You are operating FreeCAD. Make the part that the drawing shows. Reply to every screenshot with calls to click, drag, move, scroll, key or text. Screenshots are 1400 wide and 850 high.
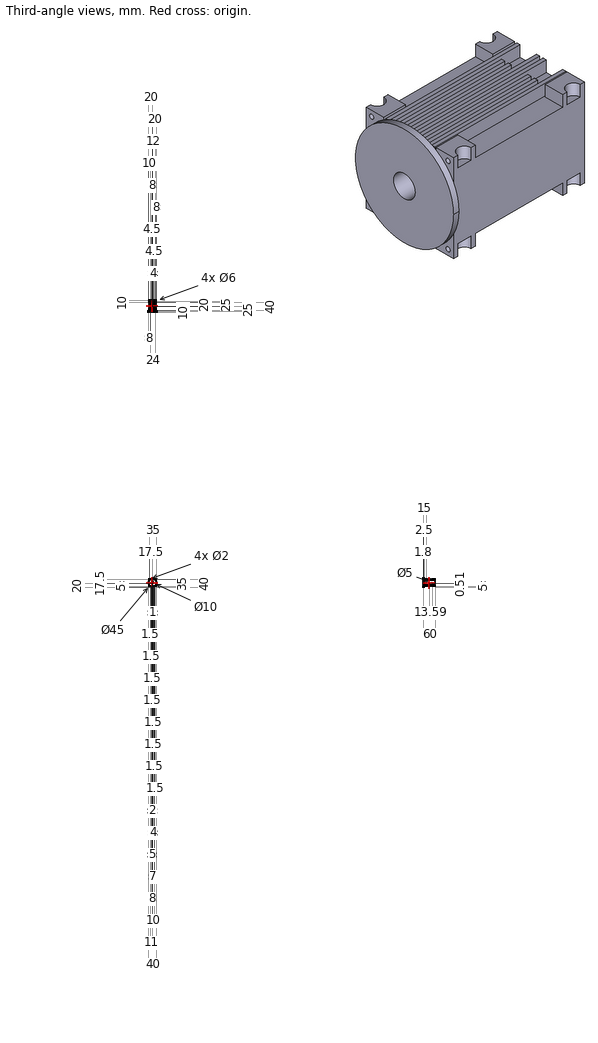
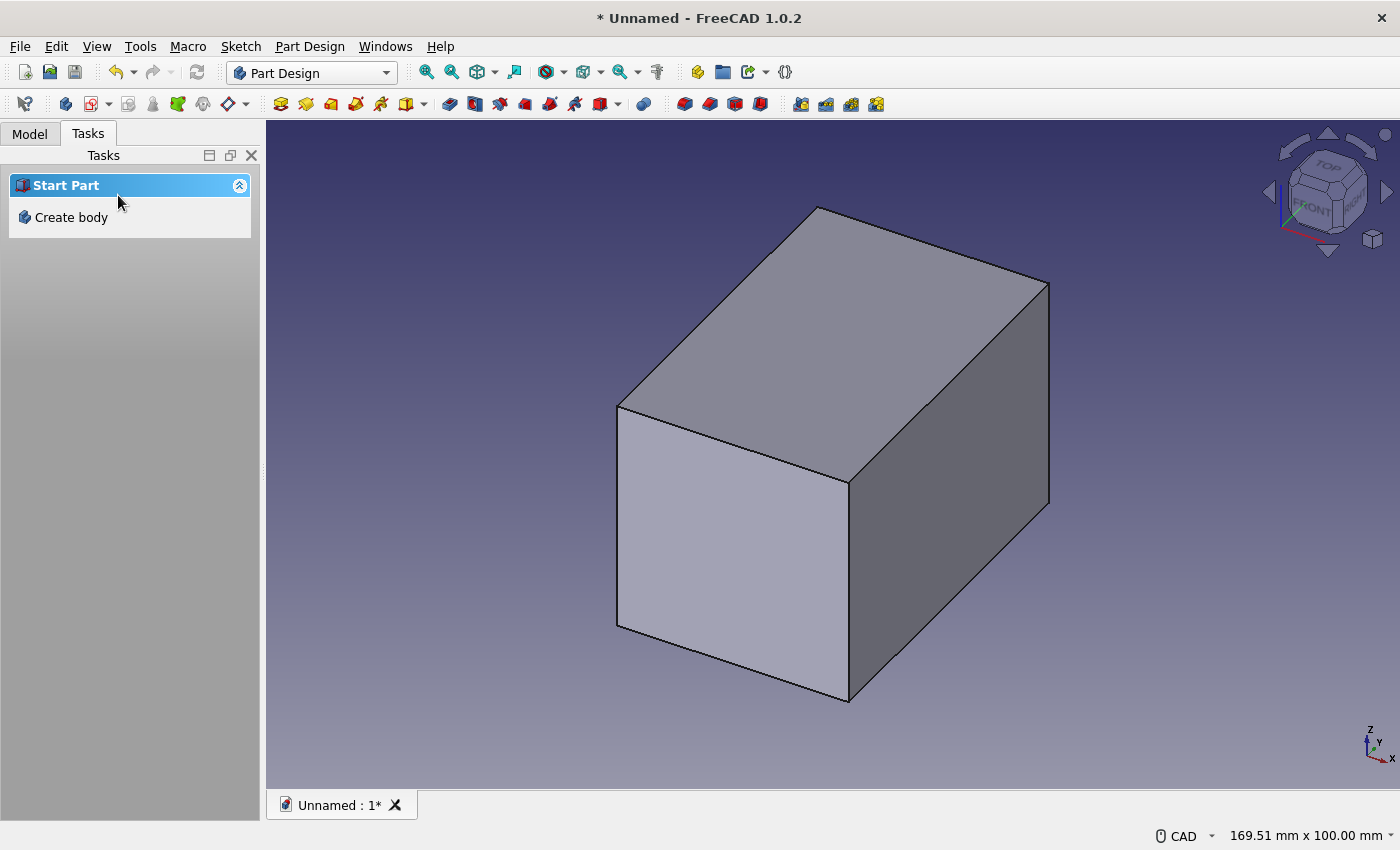
key(5)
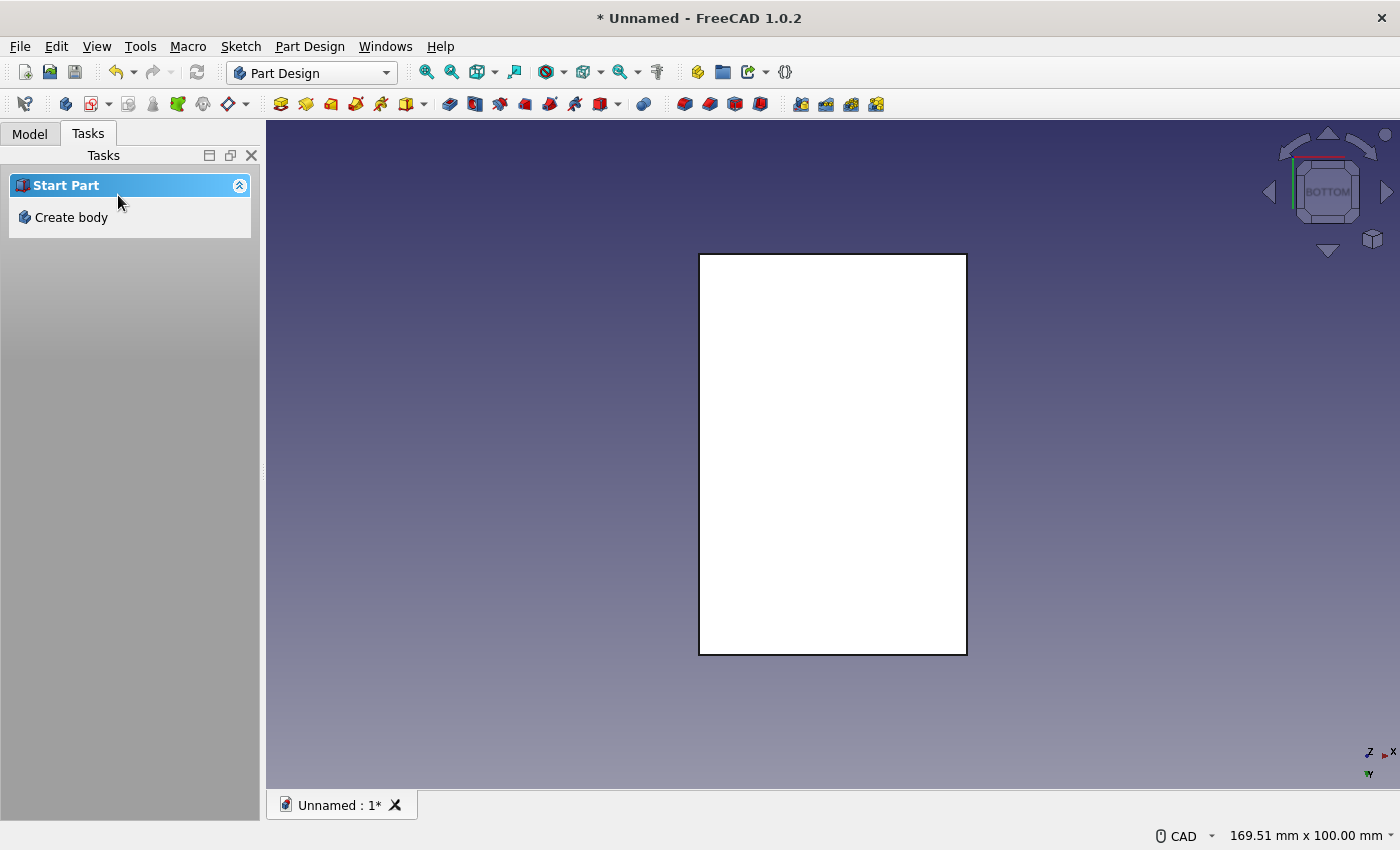
click(833, 511)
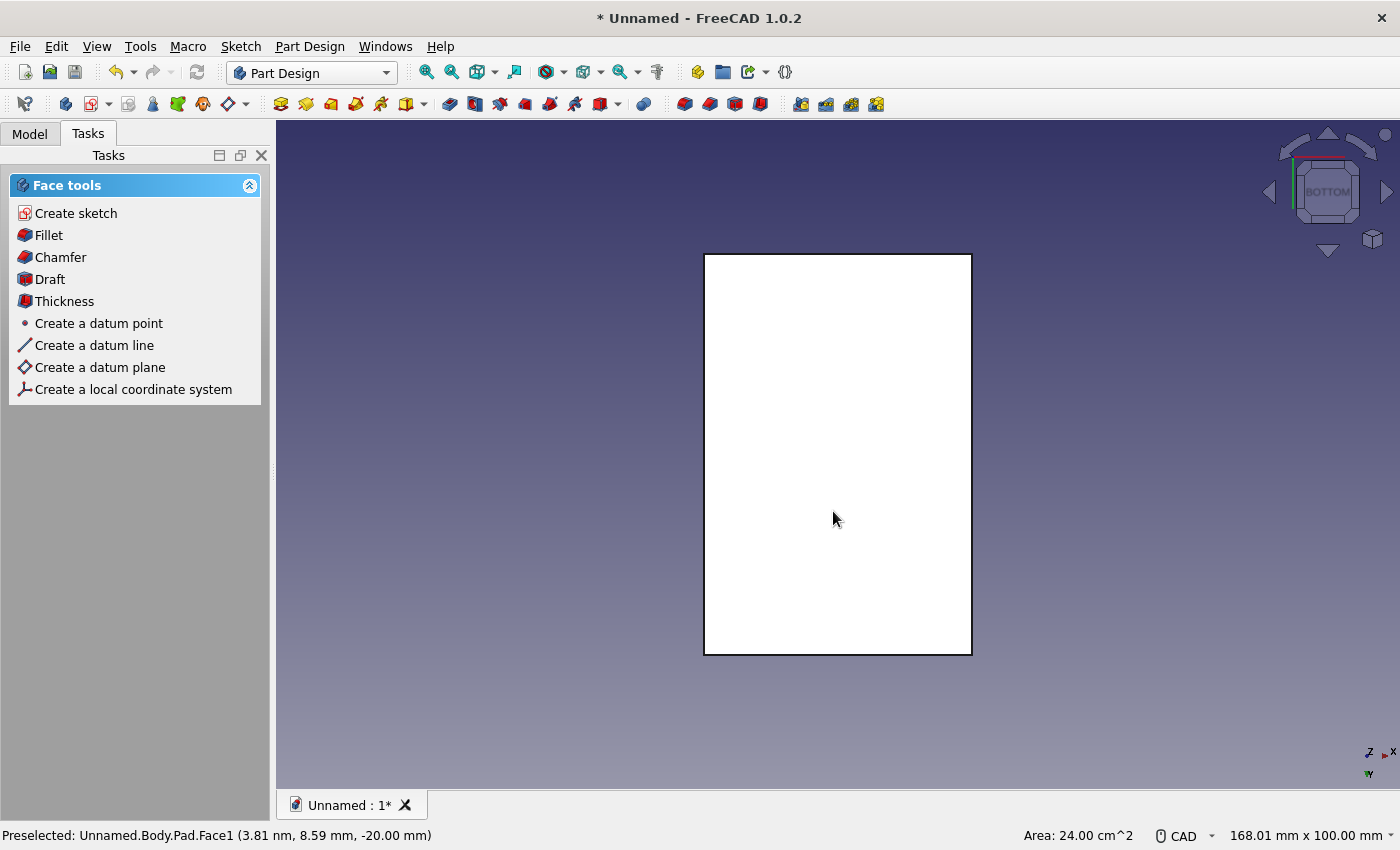
click(90, 104)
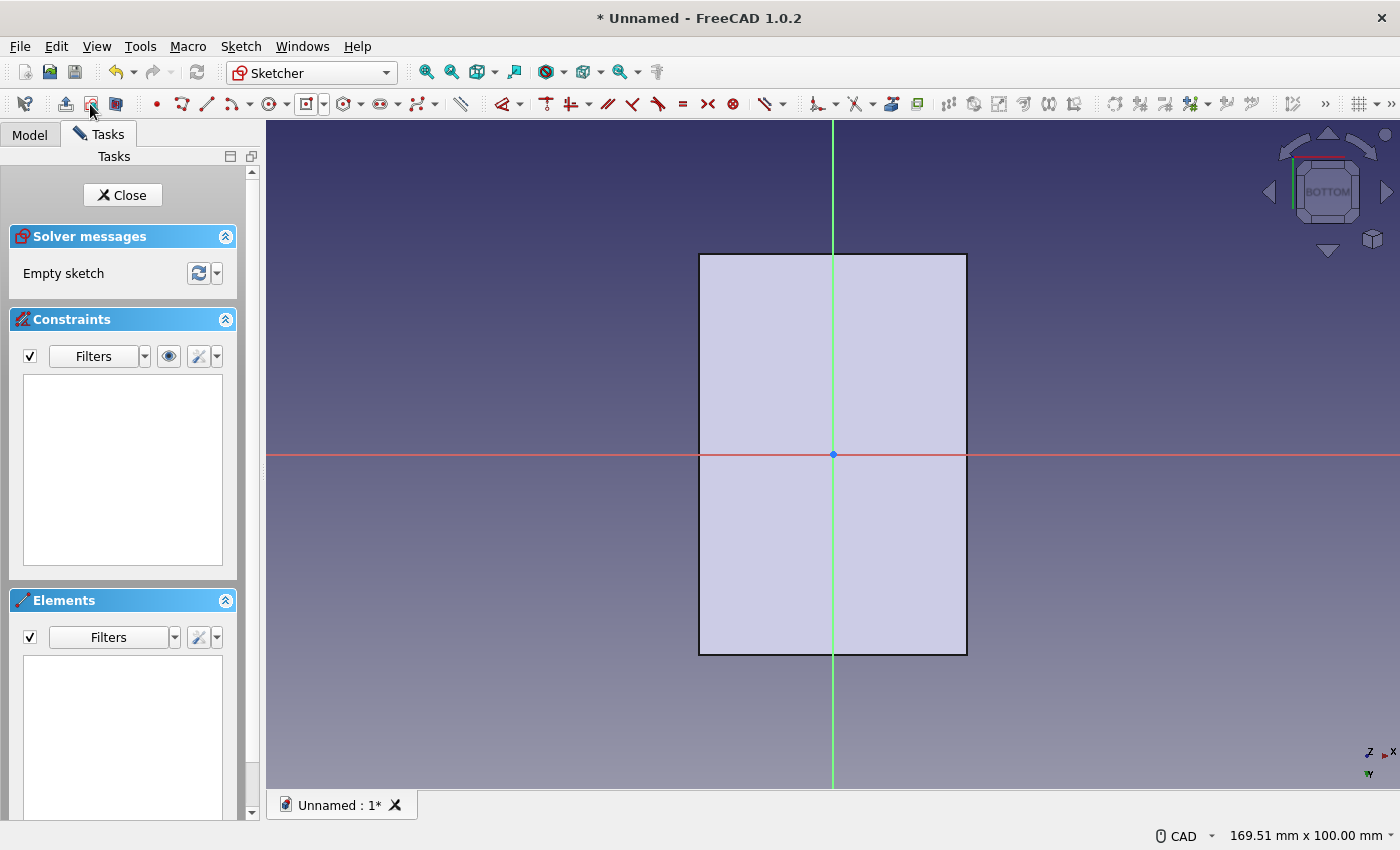
click(182, 104)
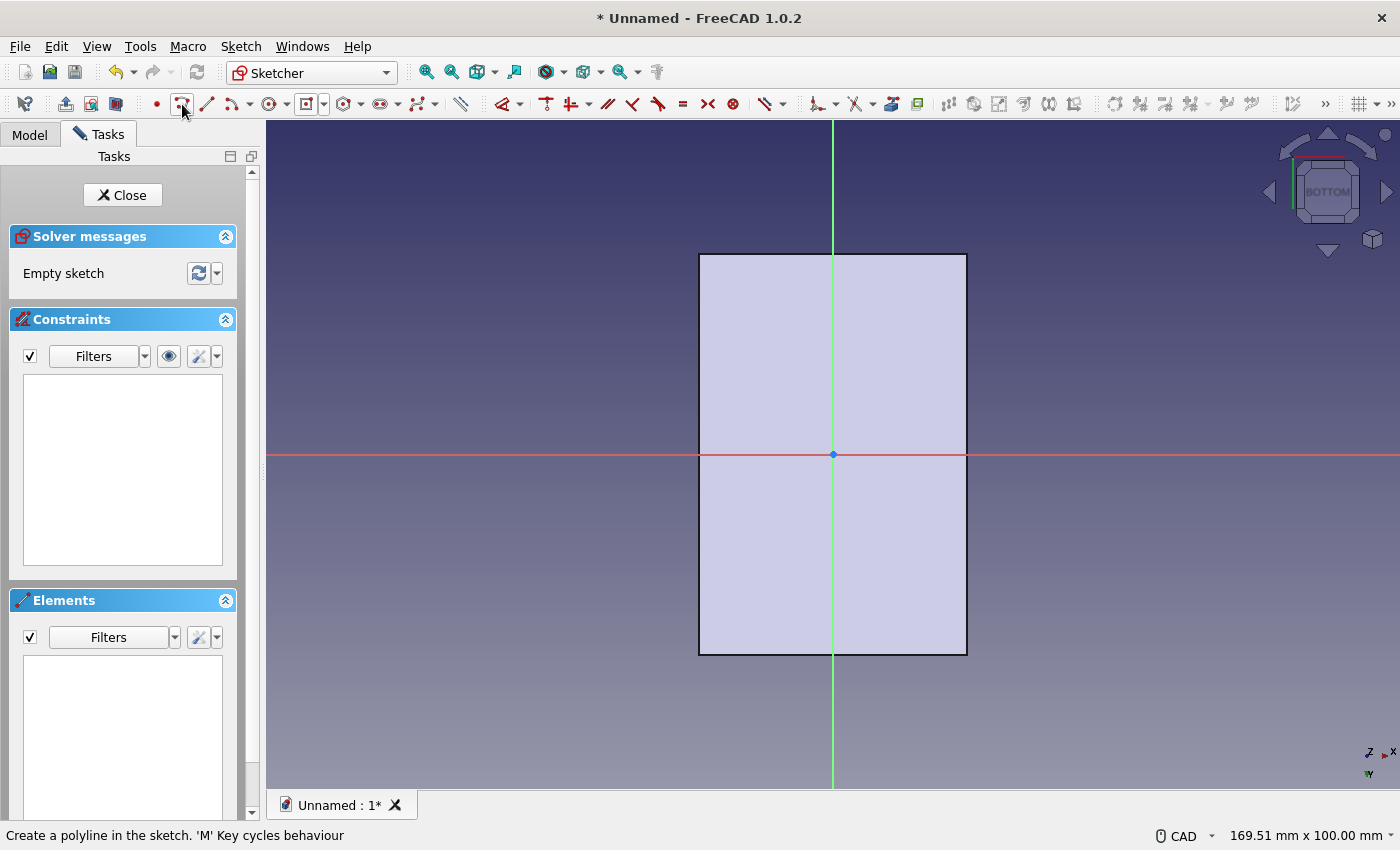
click(913, 588)
click(967, 588)
click(967, 321)
click(913, 321)
click(913, 254)
click(753, 254)
click(753, 321)
click(699, 321)
click(699, 588)
click(753, 588)
click(753, 655)
click(913, 655)
click(913, 589)
key(Escape)
key(Escape)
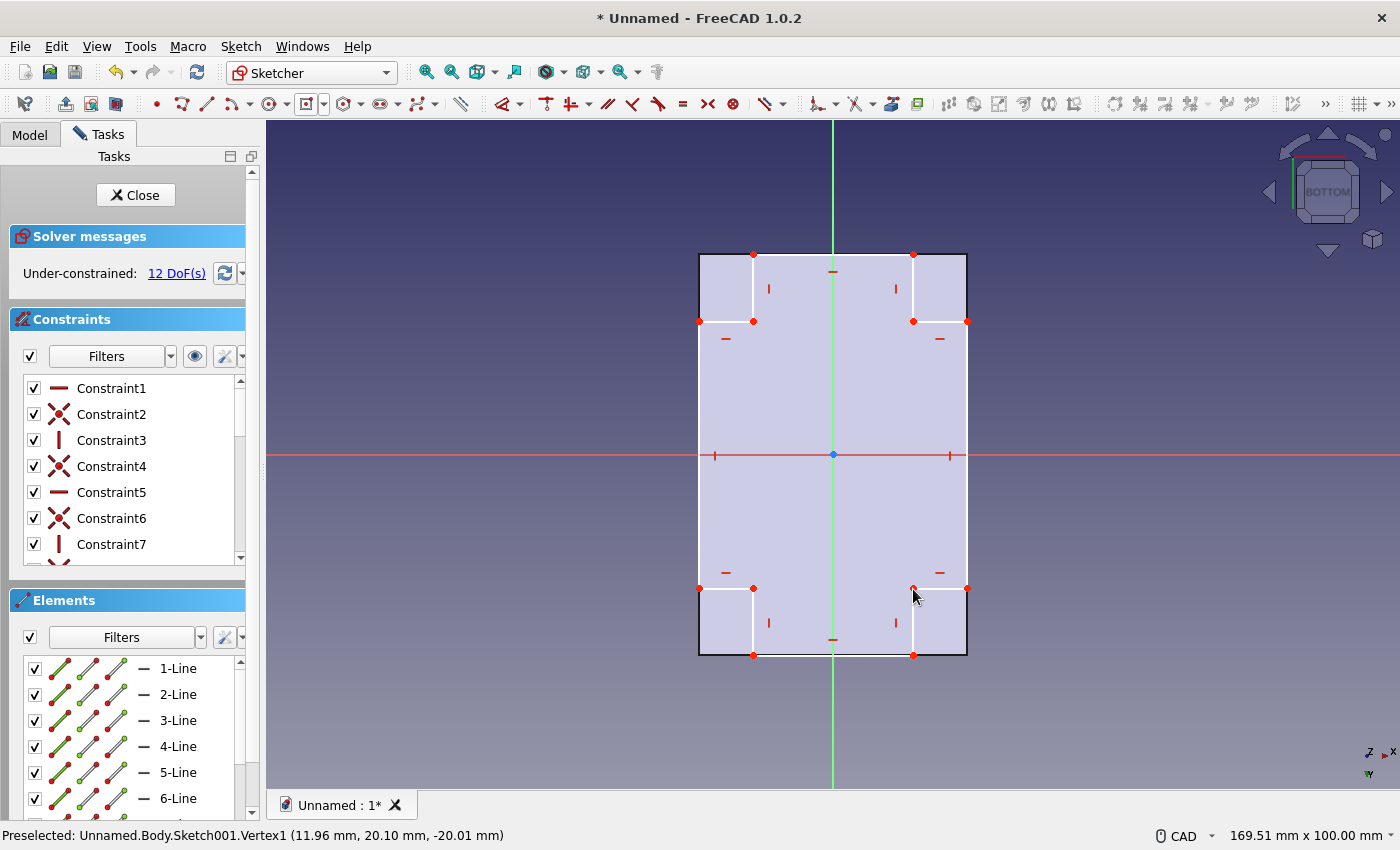
click(502, 104)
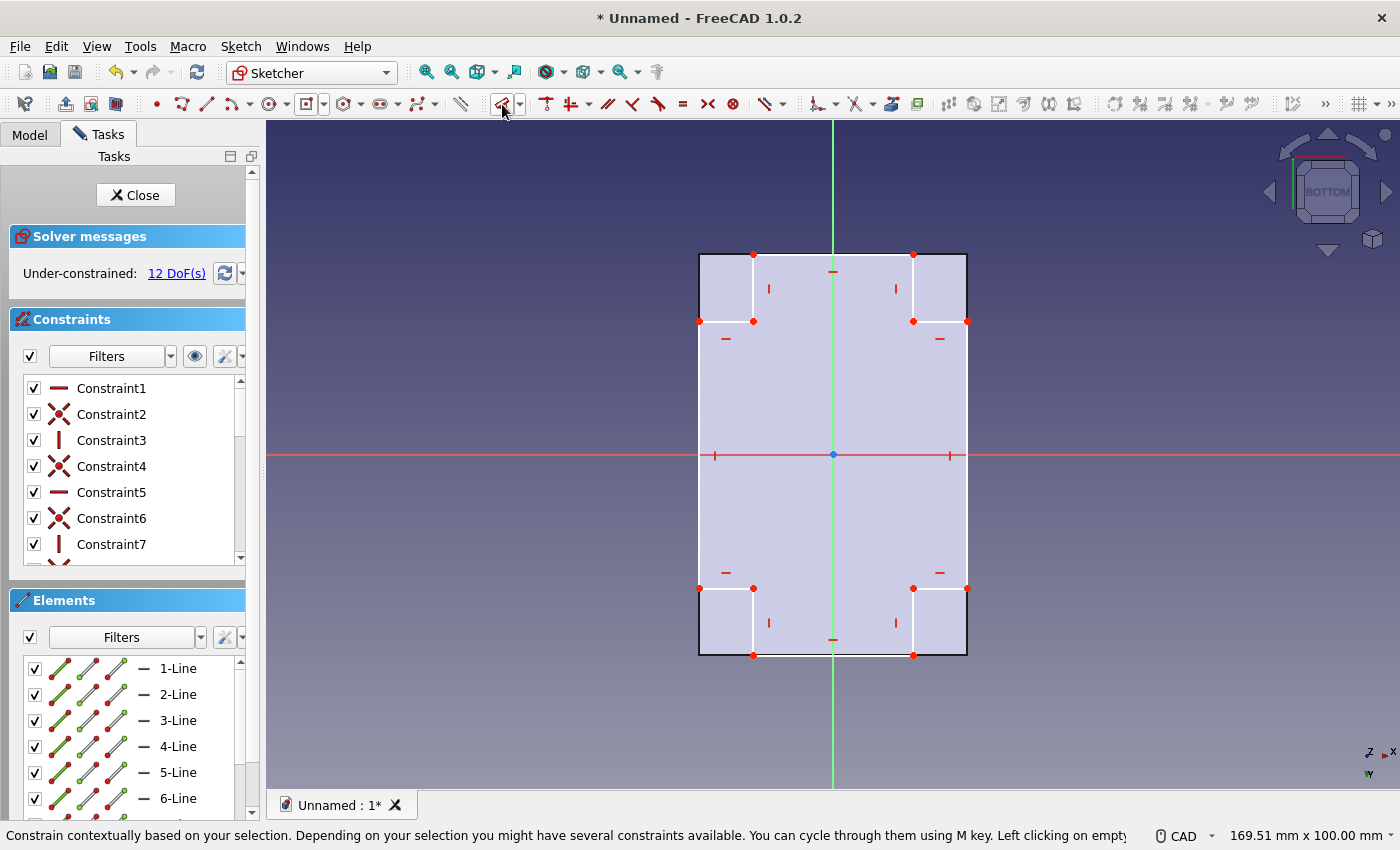
click(929, 589)
click(940, 623)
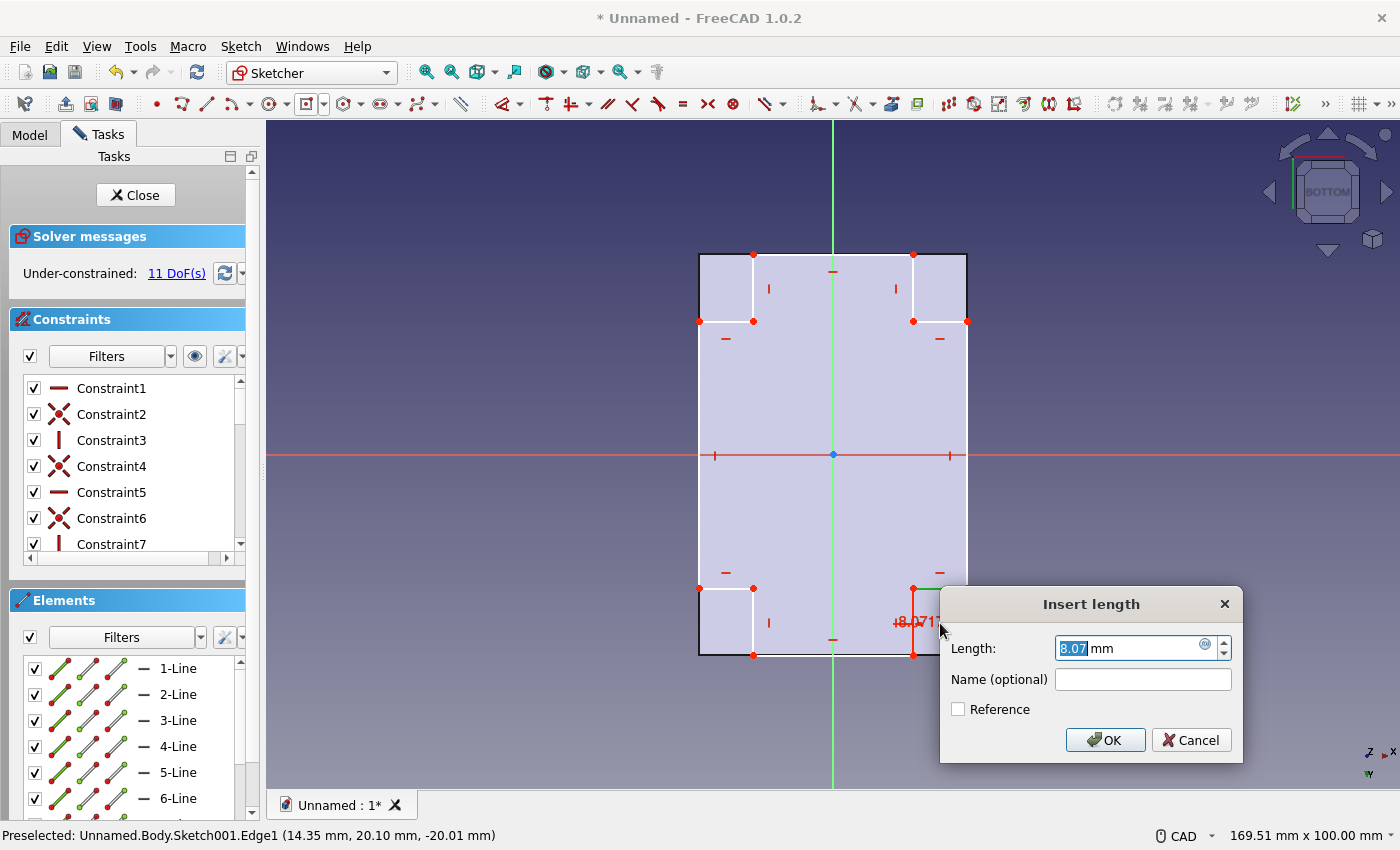
text(8)
key(Return)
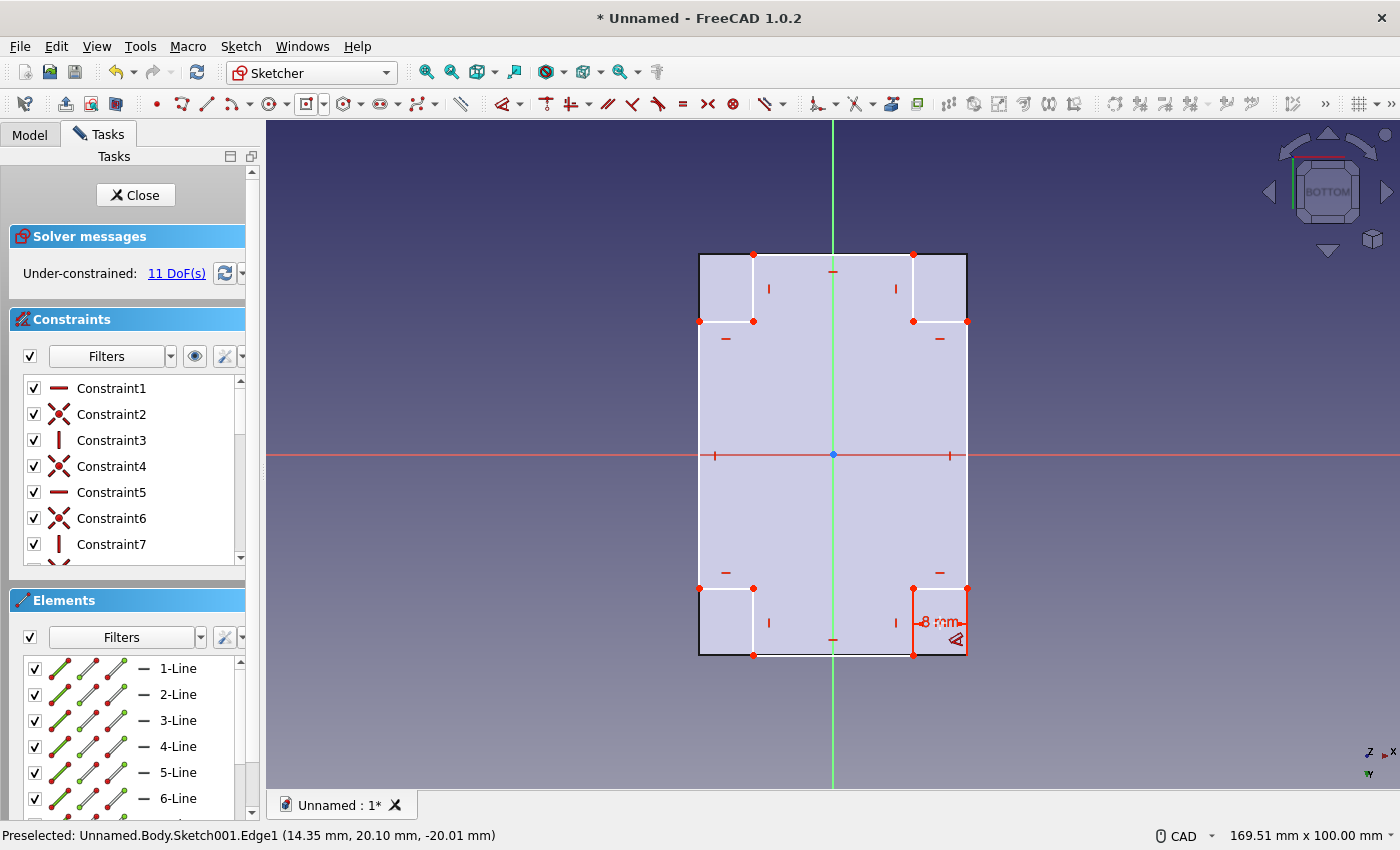
click(951, 322)
click(940, 288)